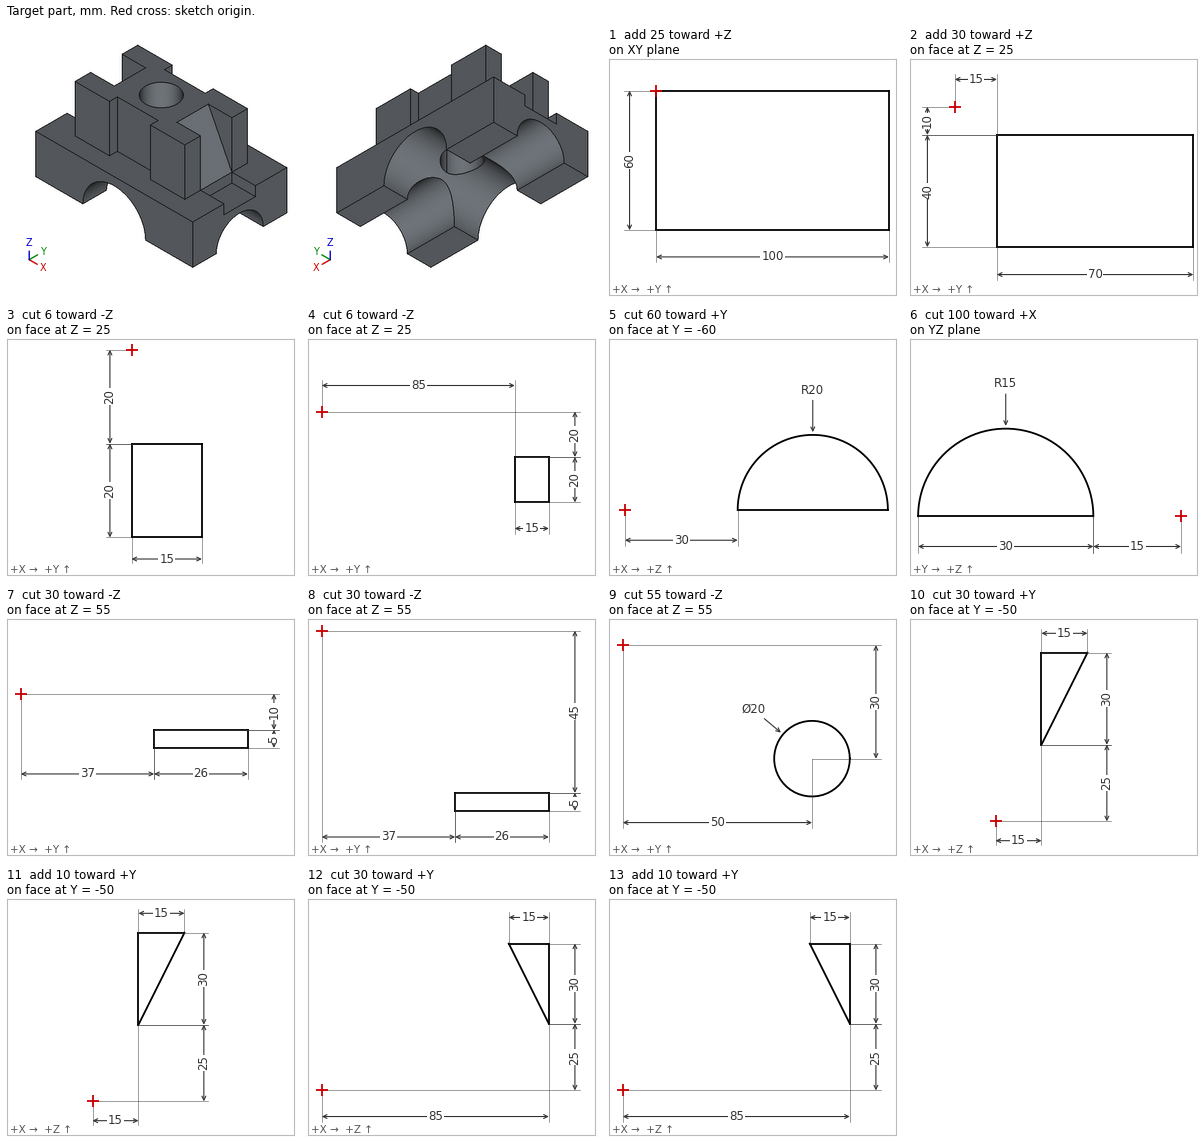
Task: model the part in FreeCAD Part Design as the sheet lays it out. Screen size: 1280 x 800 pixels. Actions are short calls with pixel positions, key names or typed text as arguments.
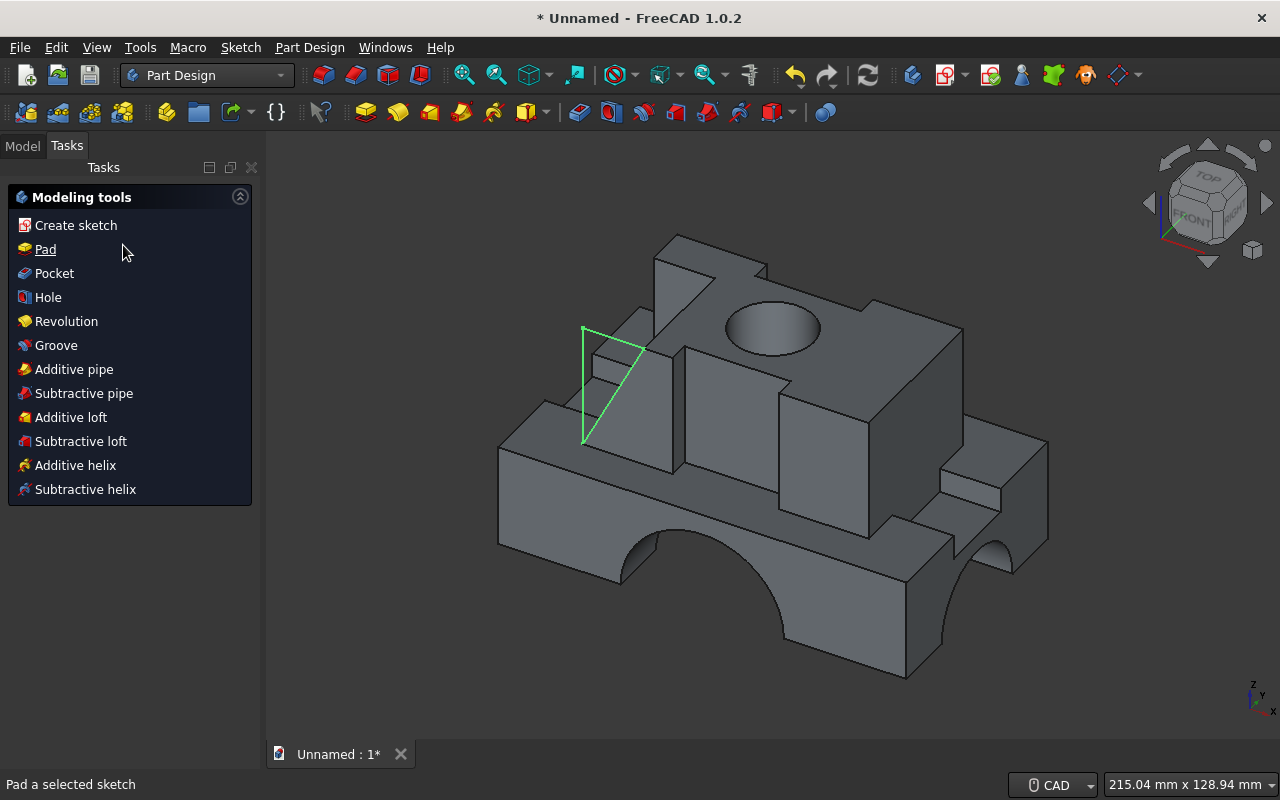
click(366, 112)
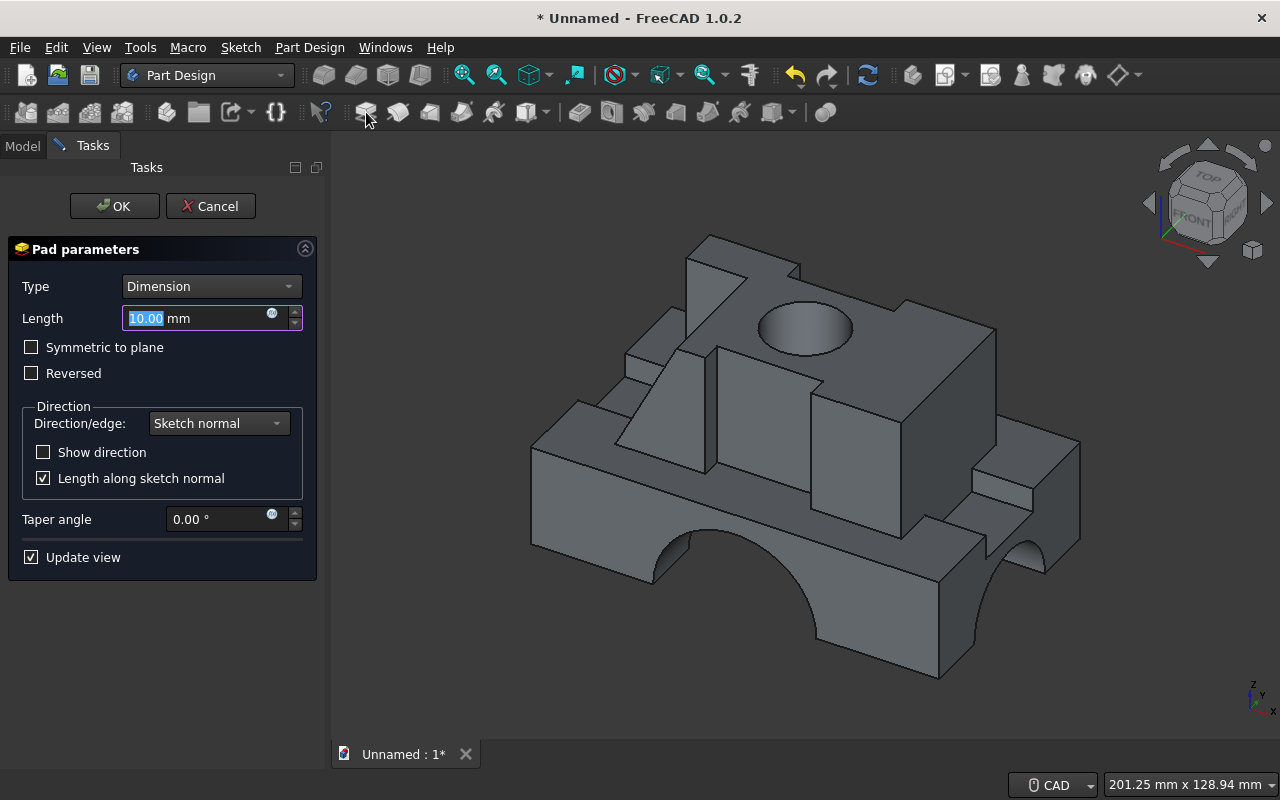
text(10)
key(Tab)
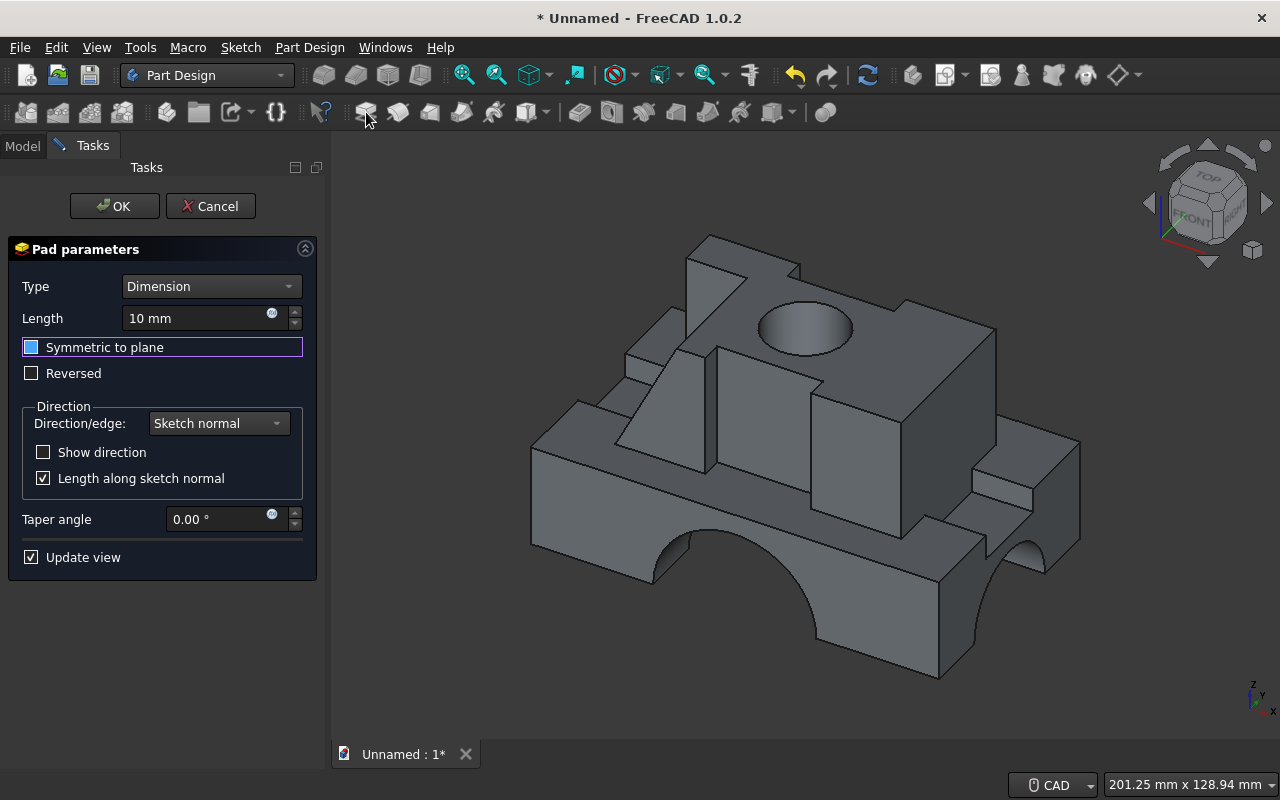
click(30, 373)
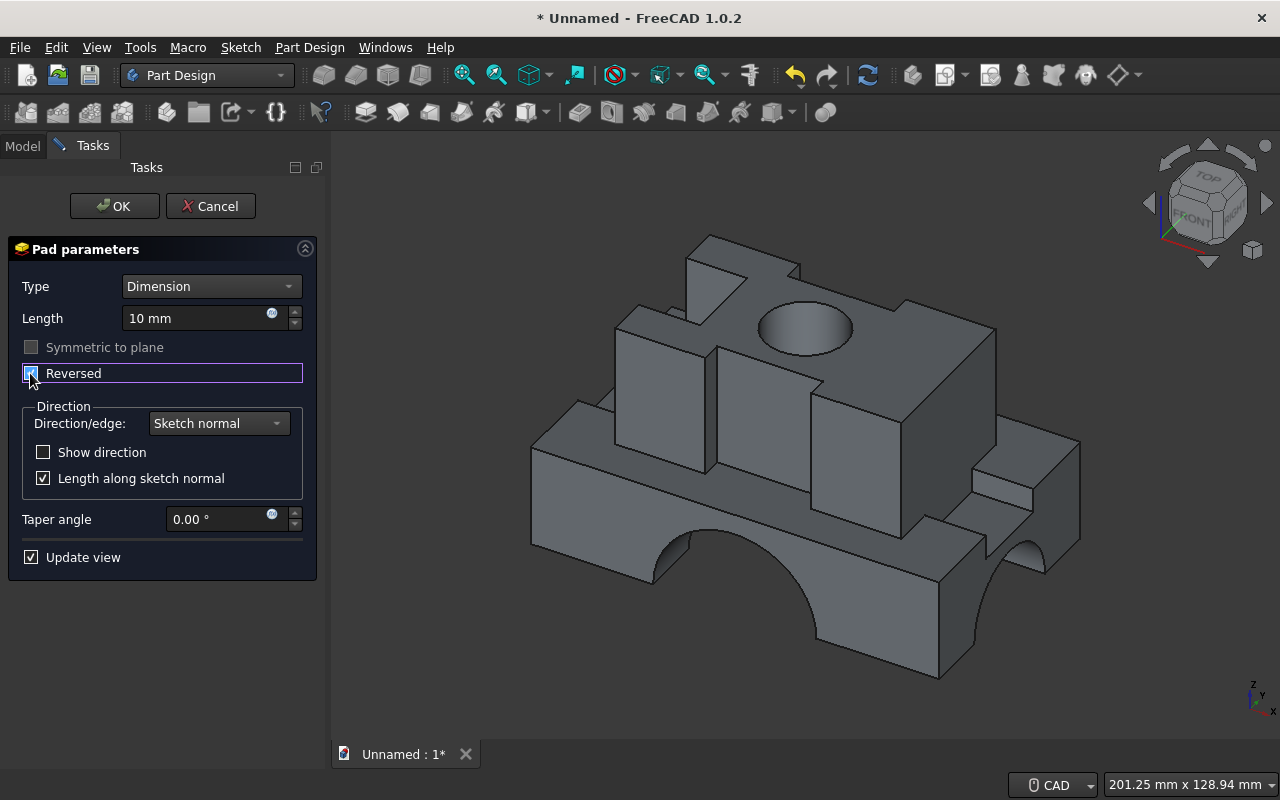
click(115, 206)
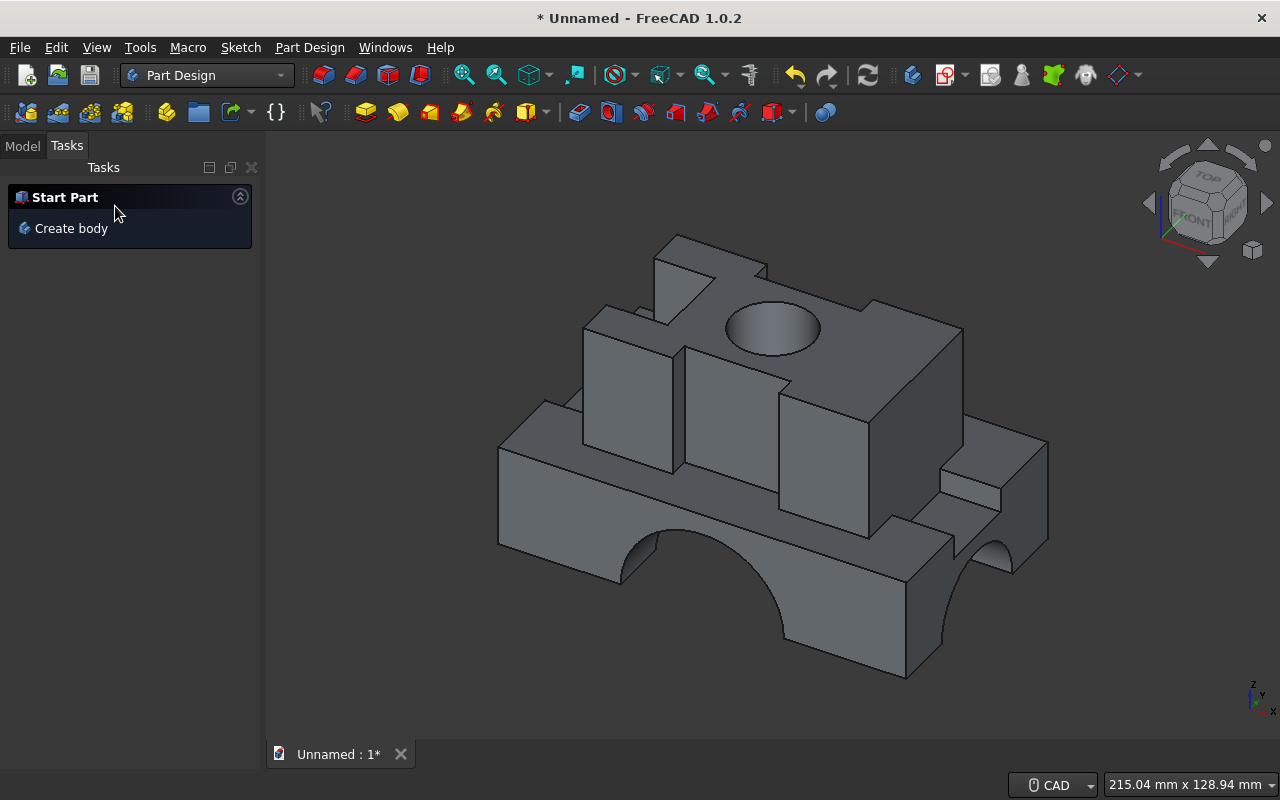
click(824, 465)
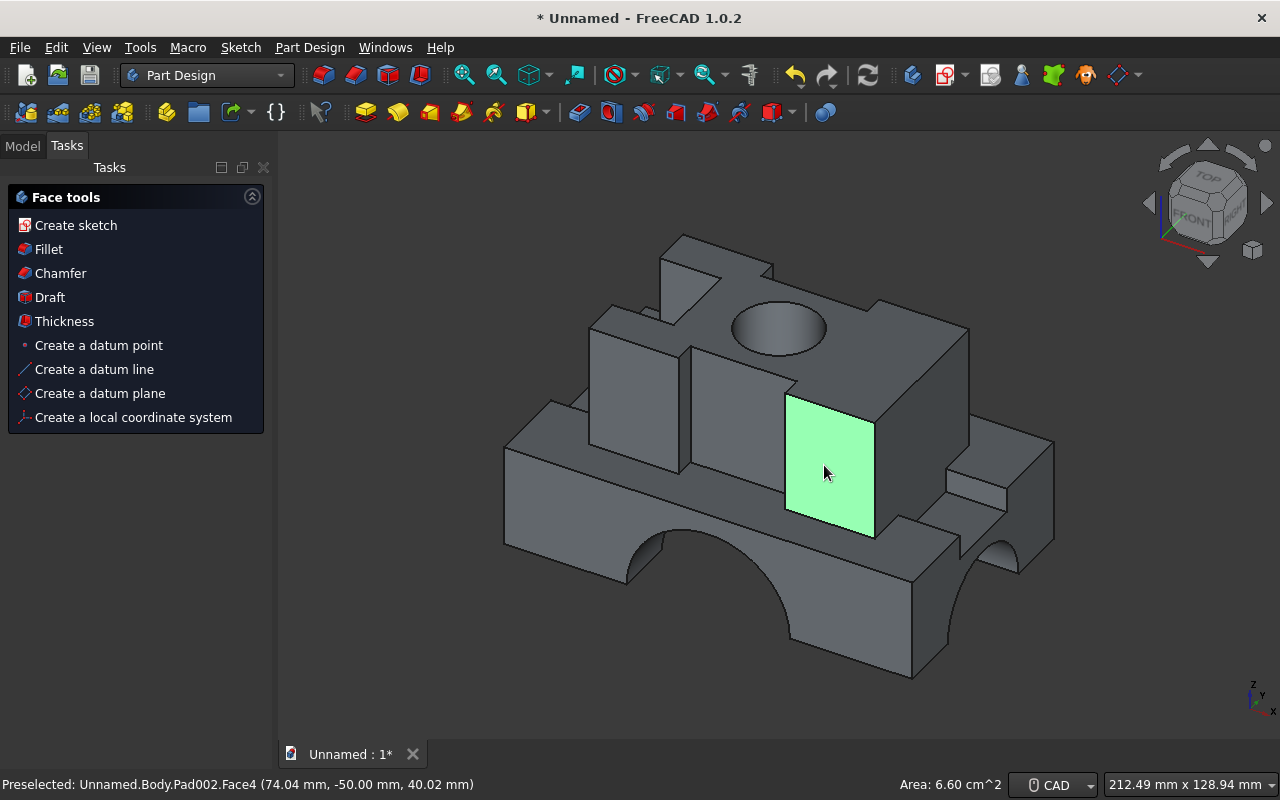
click(946, 76)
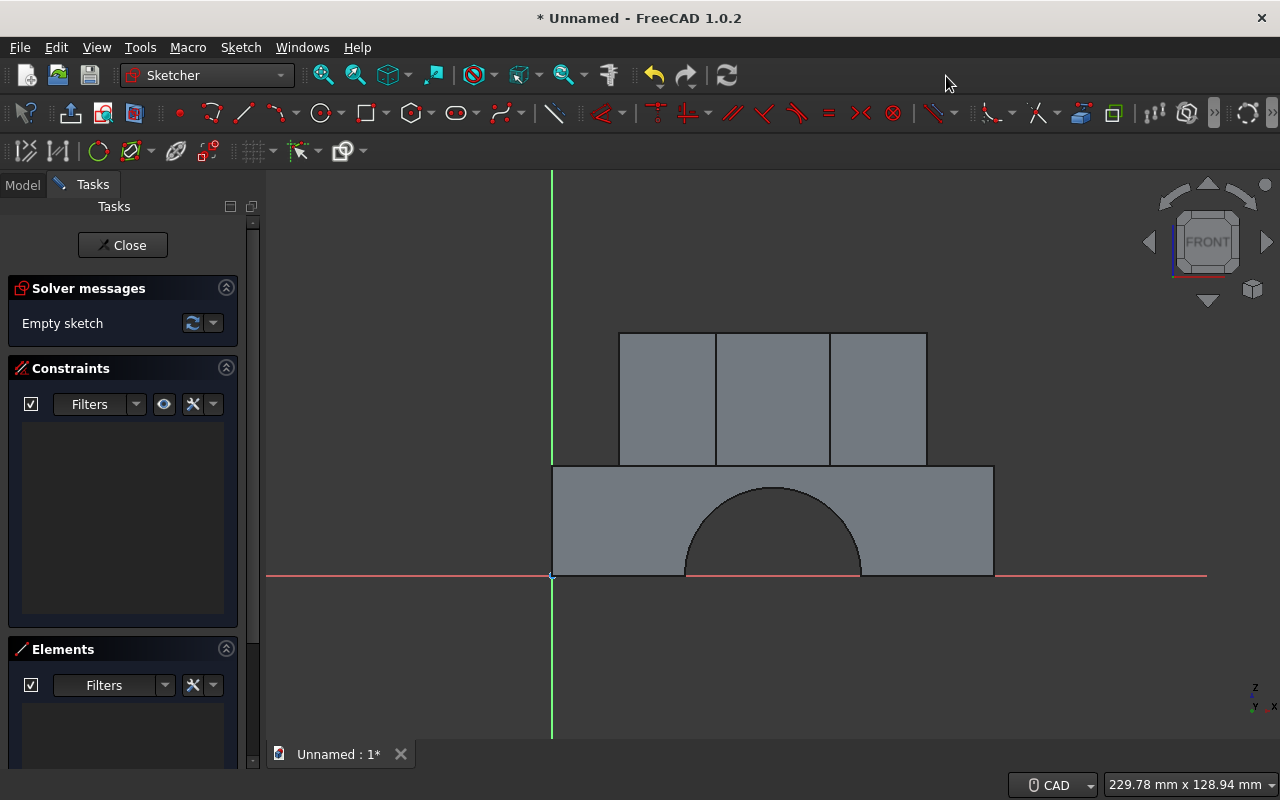
scroll(1005, 367, up, 5)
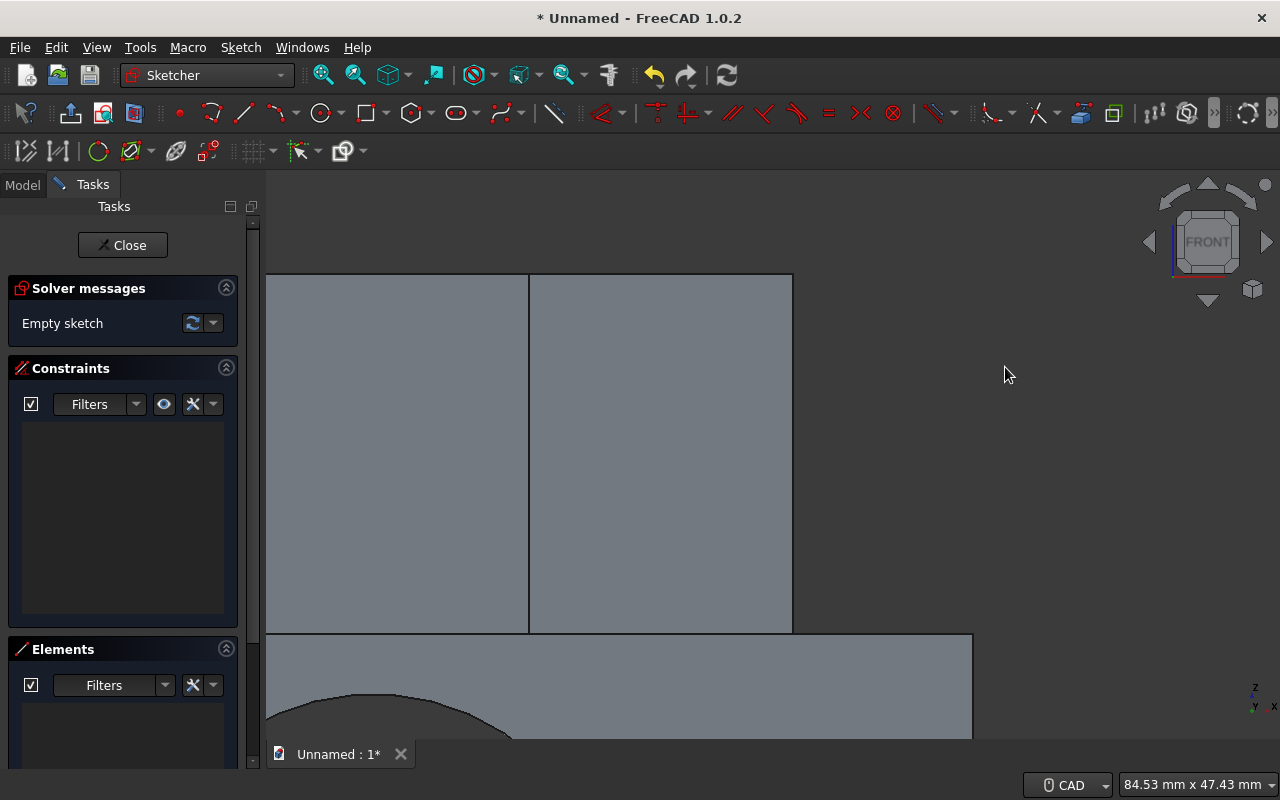
key(g)
key(m)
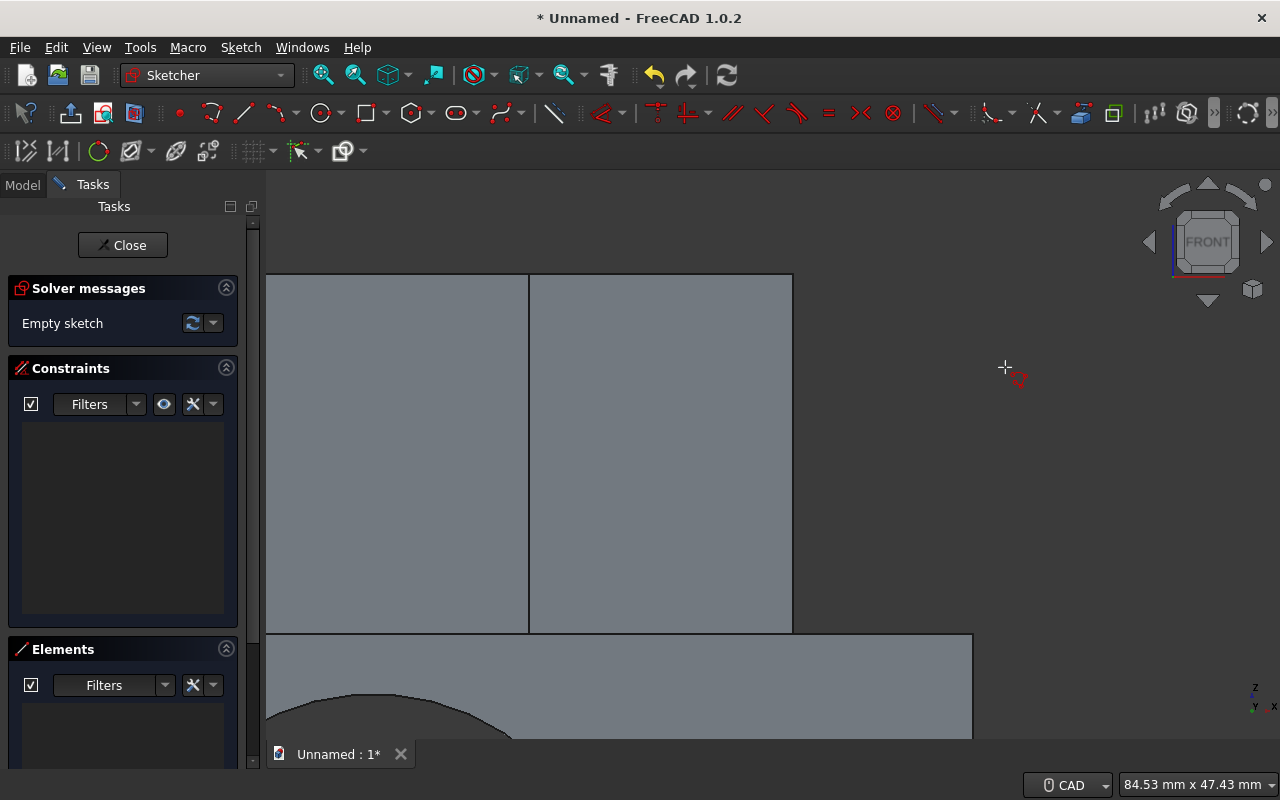
click(793, 634)
click(793, 274)
click(613, 274)
click(793, 635)
key(Escape)
key(Escape)